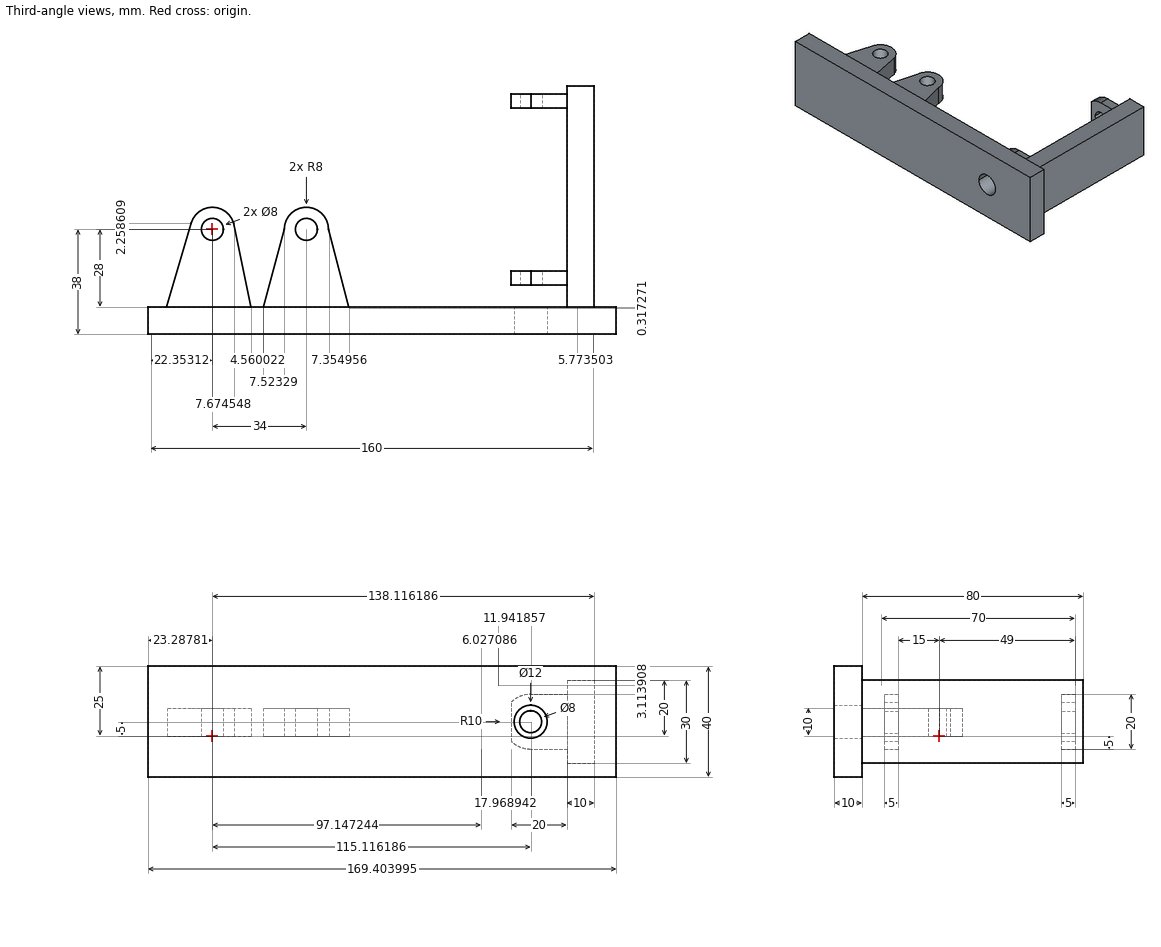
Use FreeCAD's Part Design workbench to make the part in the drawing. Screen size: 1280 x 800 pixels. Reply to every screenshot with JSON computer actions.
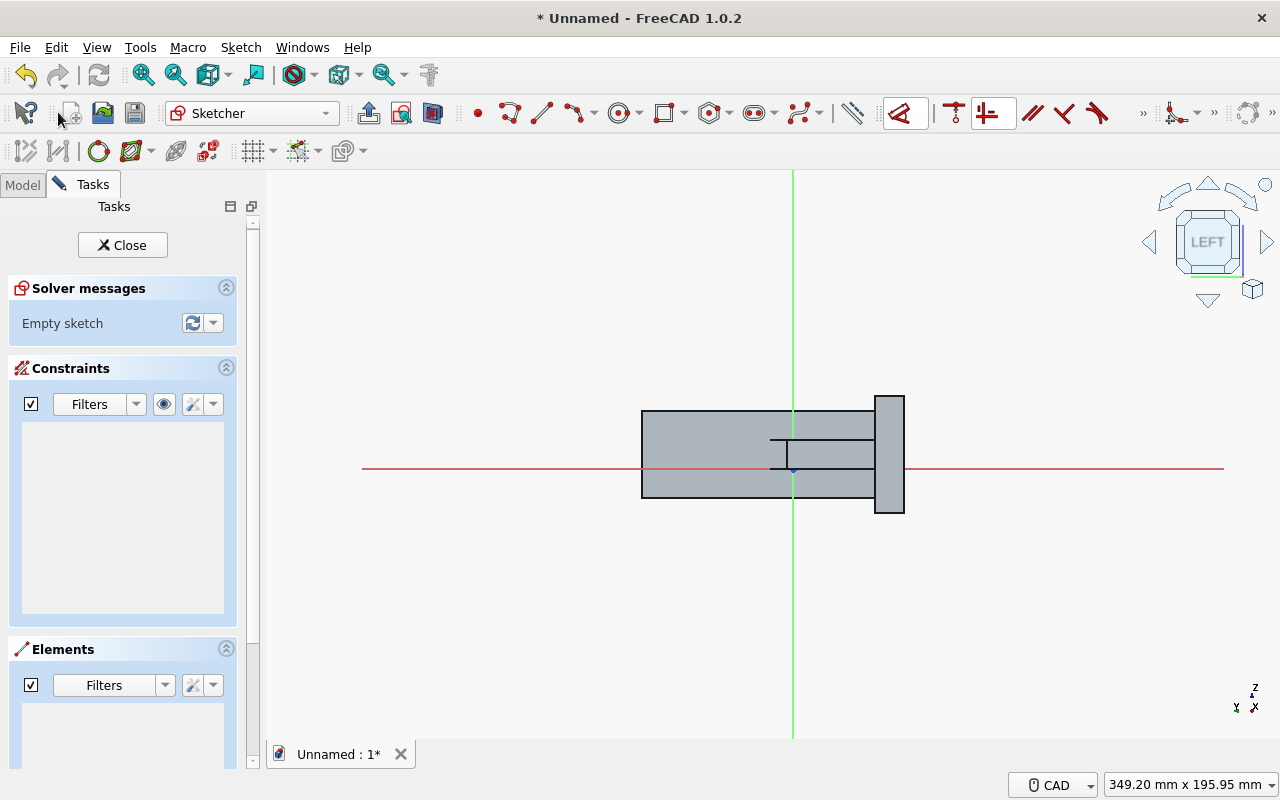
{"action": "left_click", "coordinate": [434, 114]}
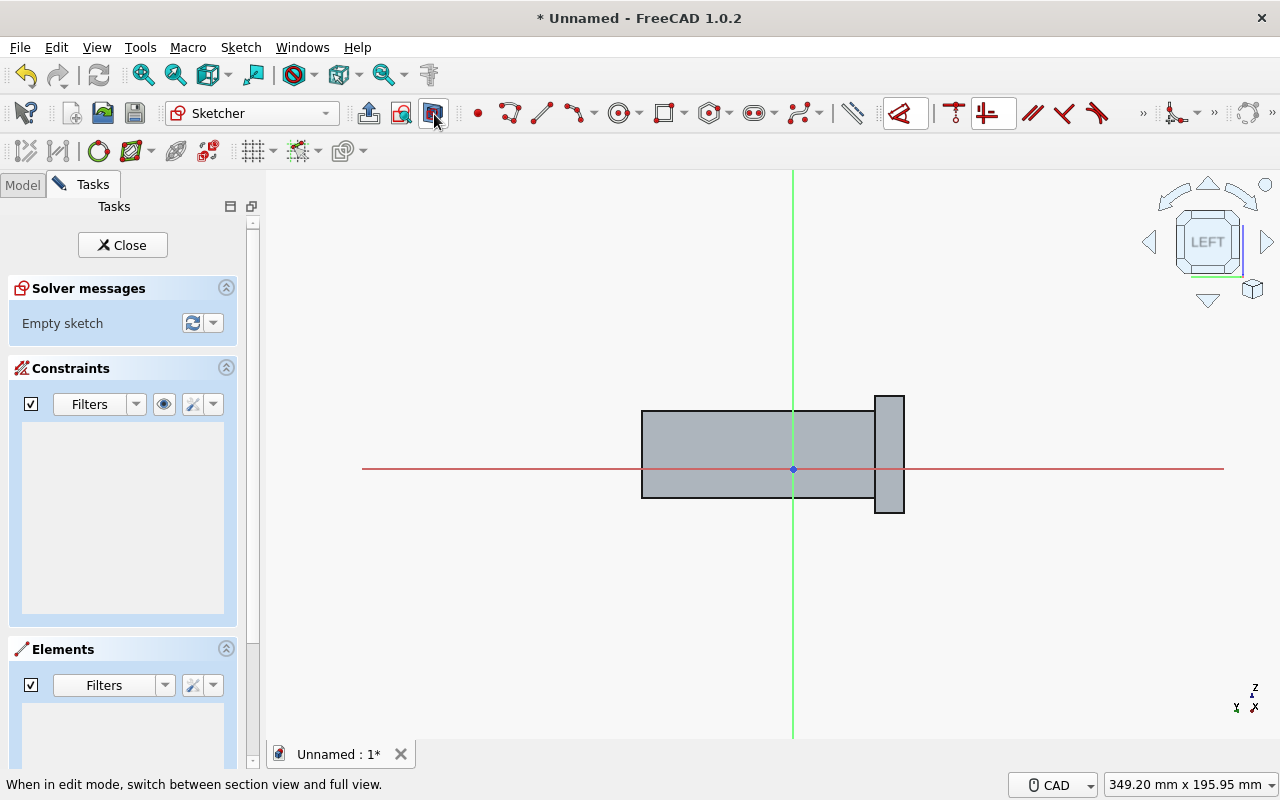
{"action": "scroll", "coordinate": [778, 454], "scroll_direction": "up", "scroll_amount": 5}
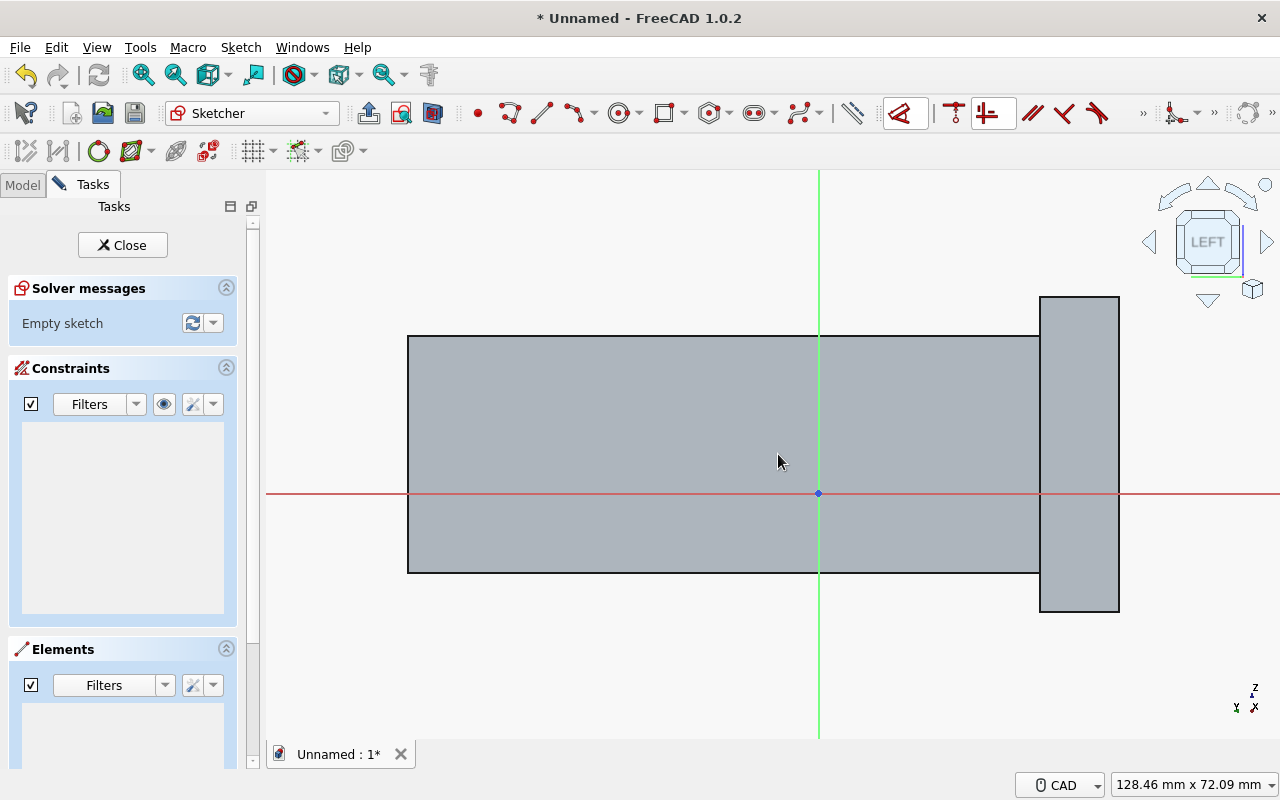
{"action": "left_click", "coordinate": [664, 114]}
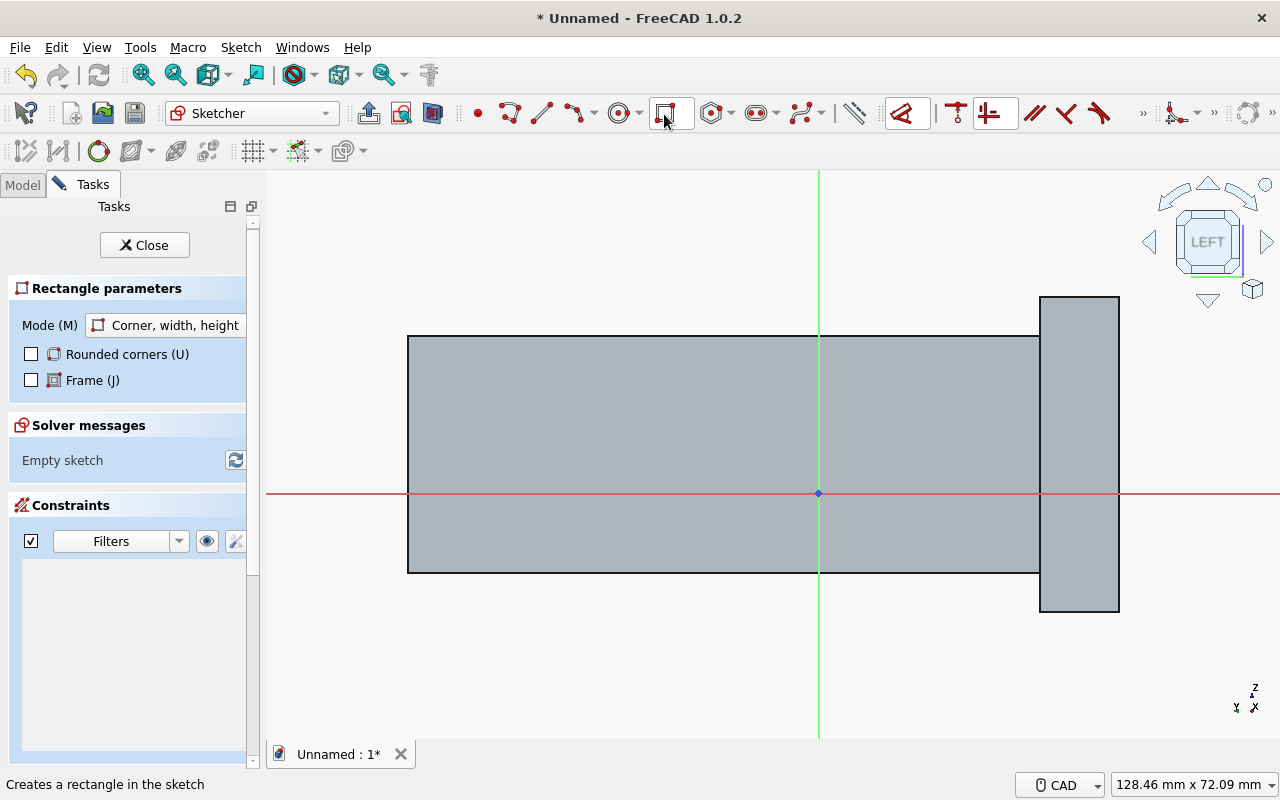
{"action": "left_click", "coordinate": [432, 376]}
{"action": "mouse_move", "coordinate": [471, 533]}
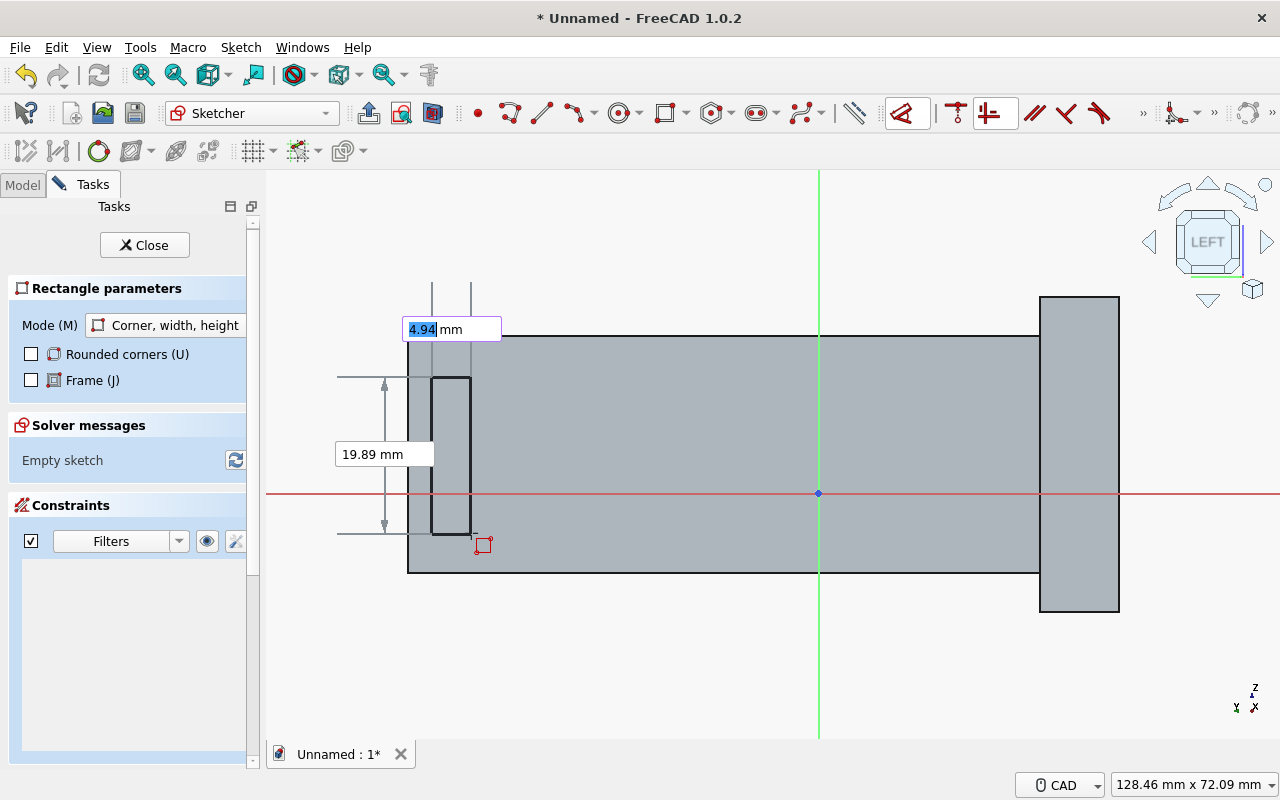
{"action": "type", "text": "5"}
{"action": "key", "text": "Tab"}
{"action": "type", "text": "20"}
{"action": "key", "text": "Return"}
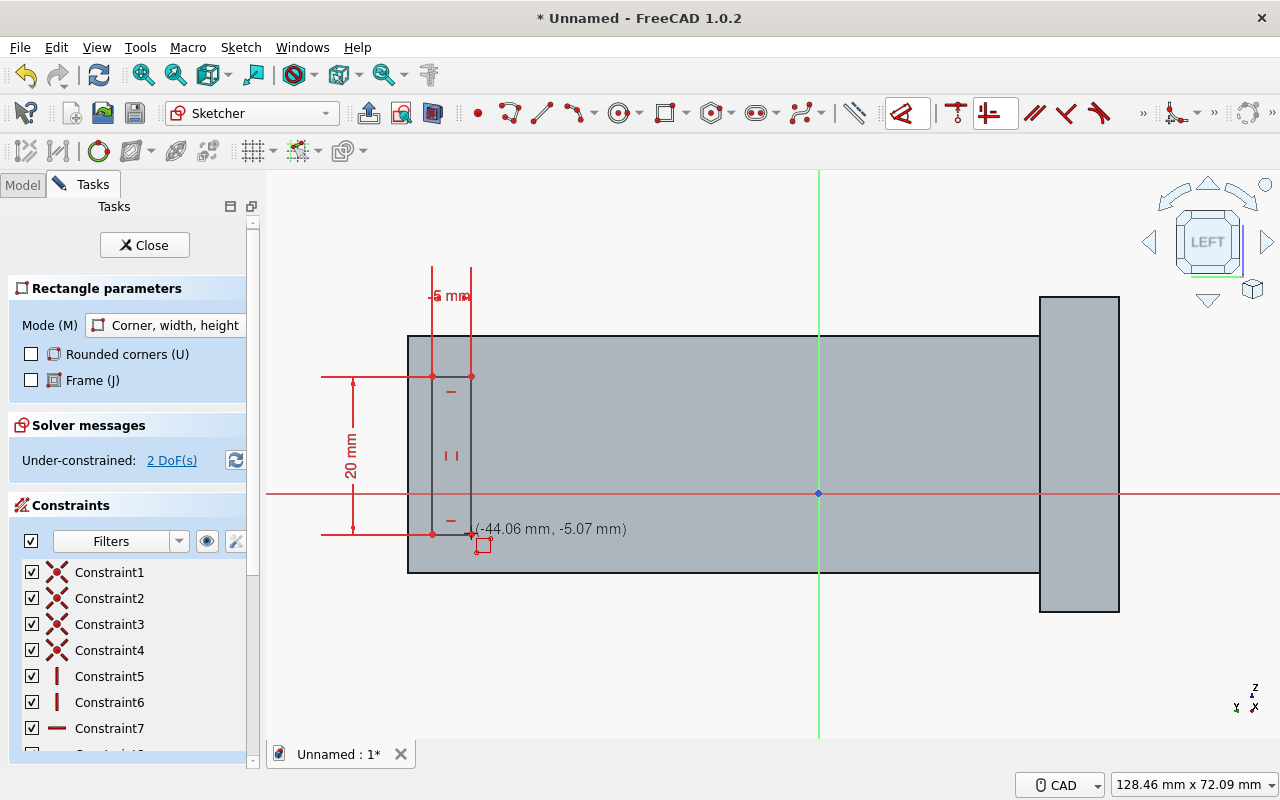
{"action": "left_click", "coordinate": [937, 376]}
{"action": "mouse_move", "coordinate": [977, 533]}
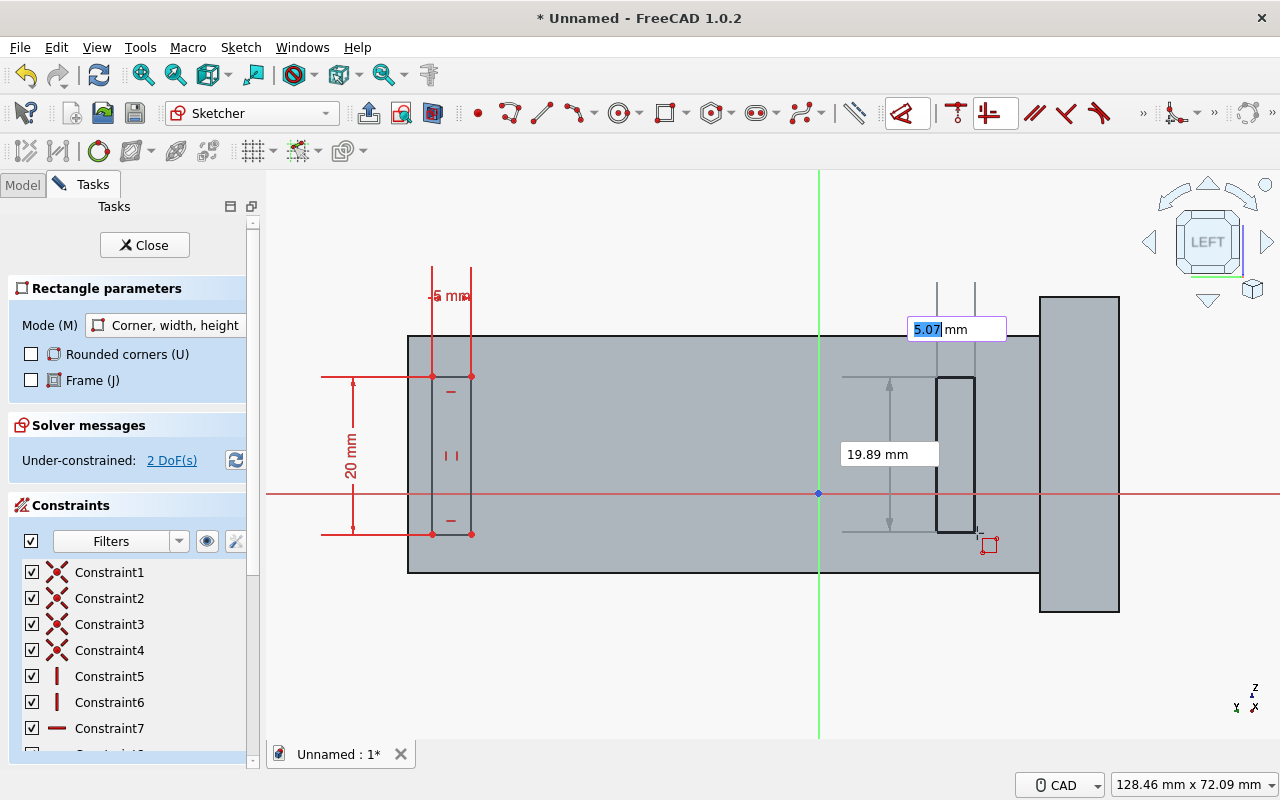
{"action": "type", "text": "5"}
{"action": "key", "text": "Tab"}
{"action": "type", "text": "20"}
{"action": "key", "text": "Return"}
{"action": "key", "text": "Escape"}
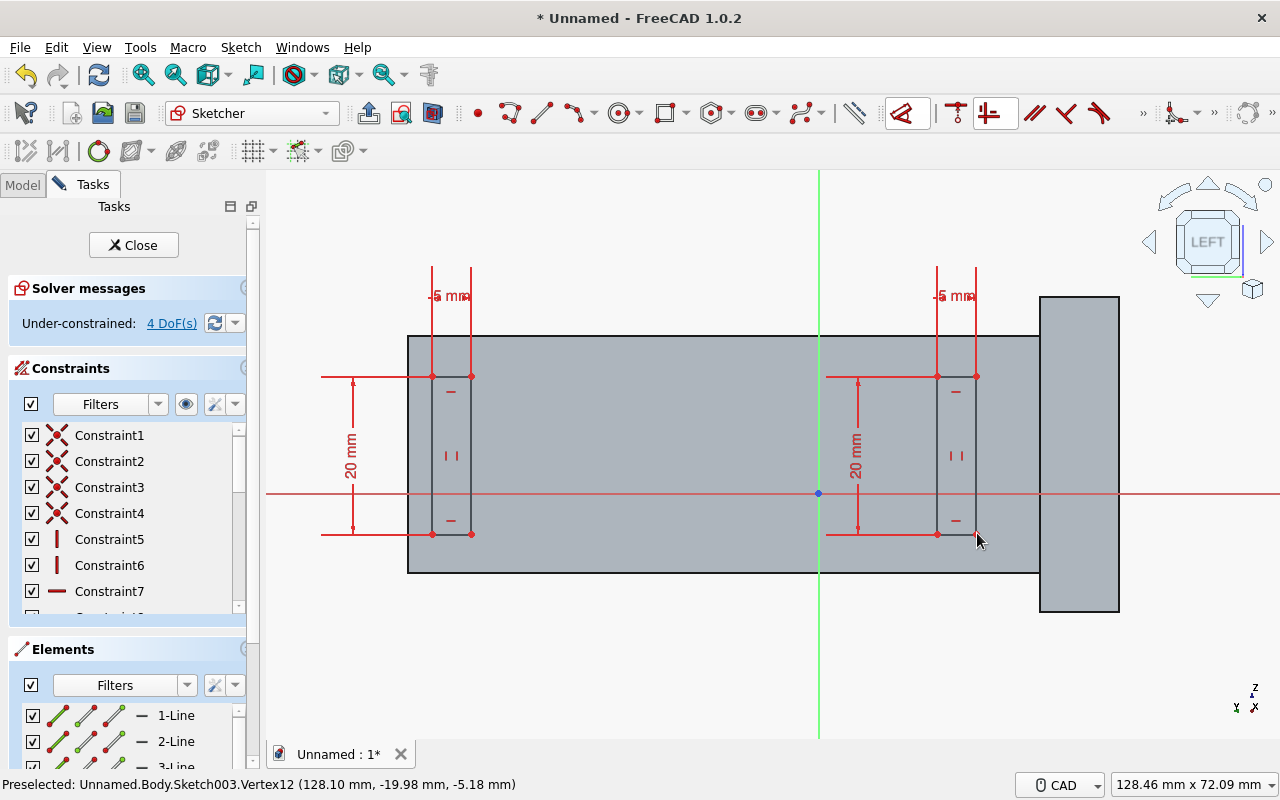
{"action": "left_click", "coordinate": [432, 535]}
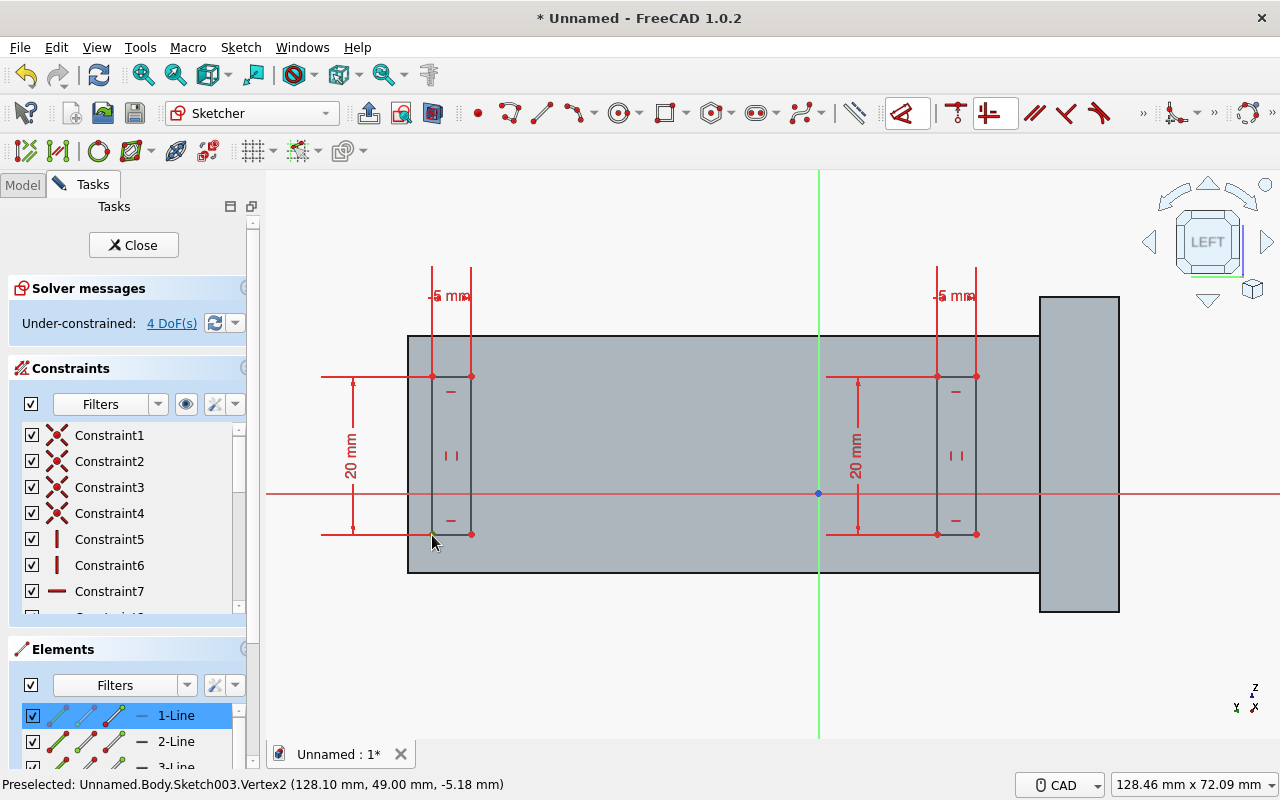
{"action": "key", "text": "i"}